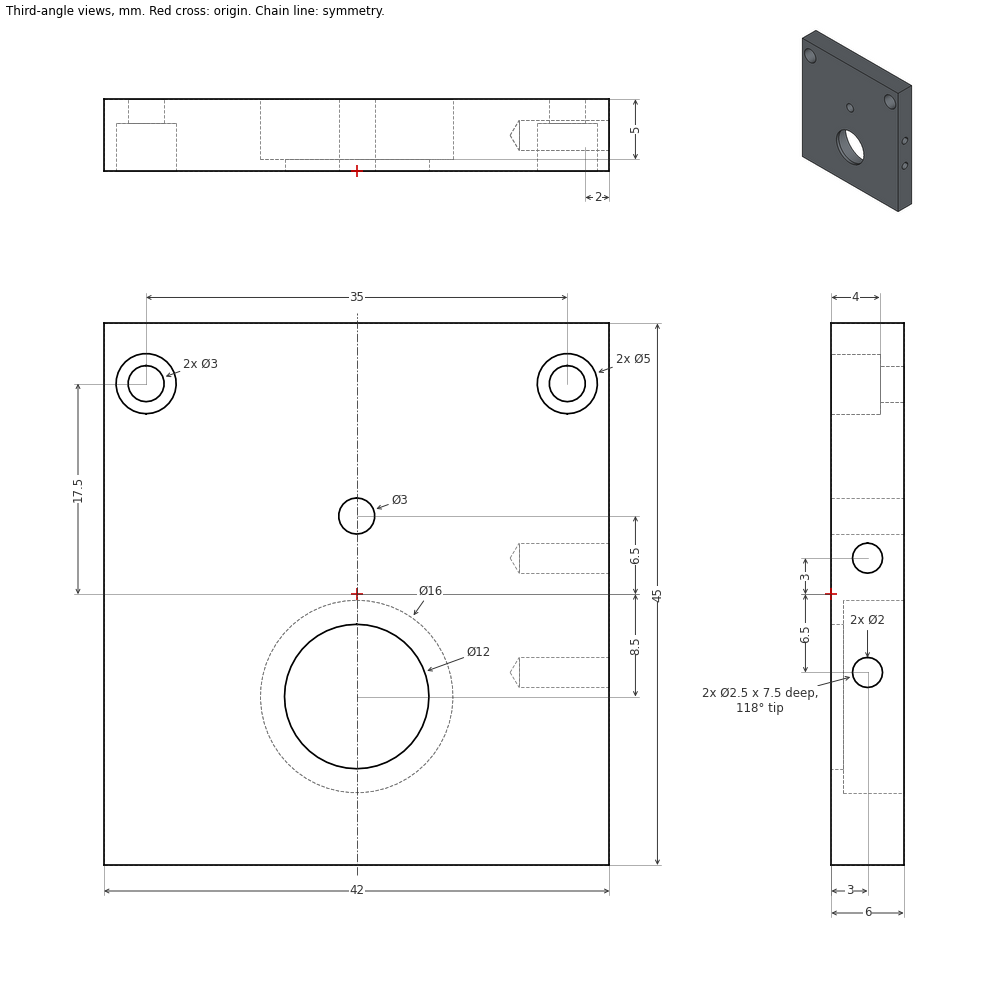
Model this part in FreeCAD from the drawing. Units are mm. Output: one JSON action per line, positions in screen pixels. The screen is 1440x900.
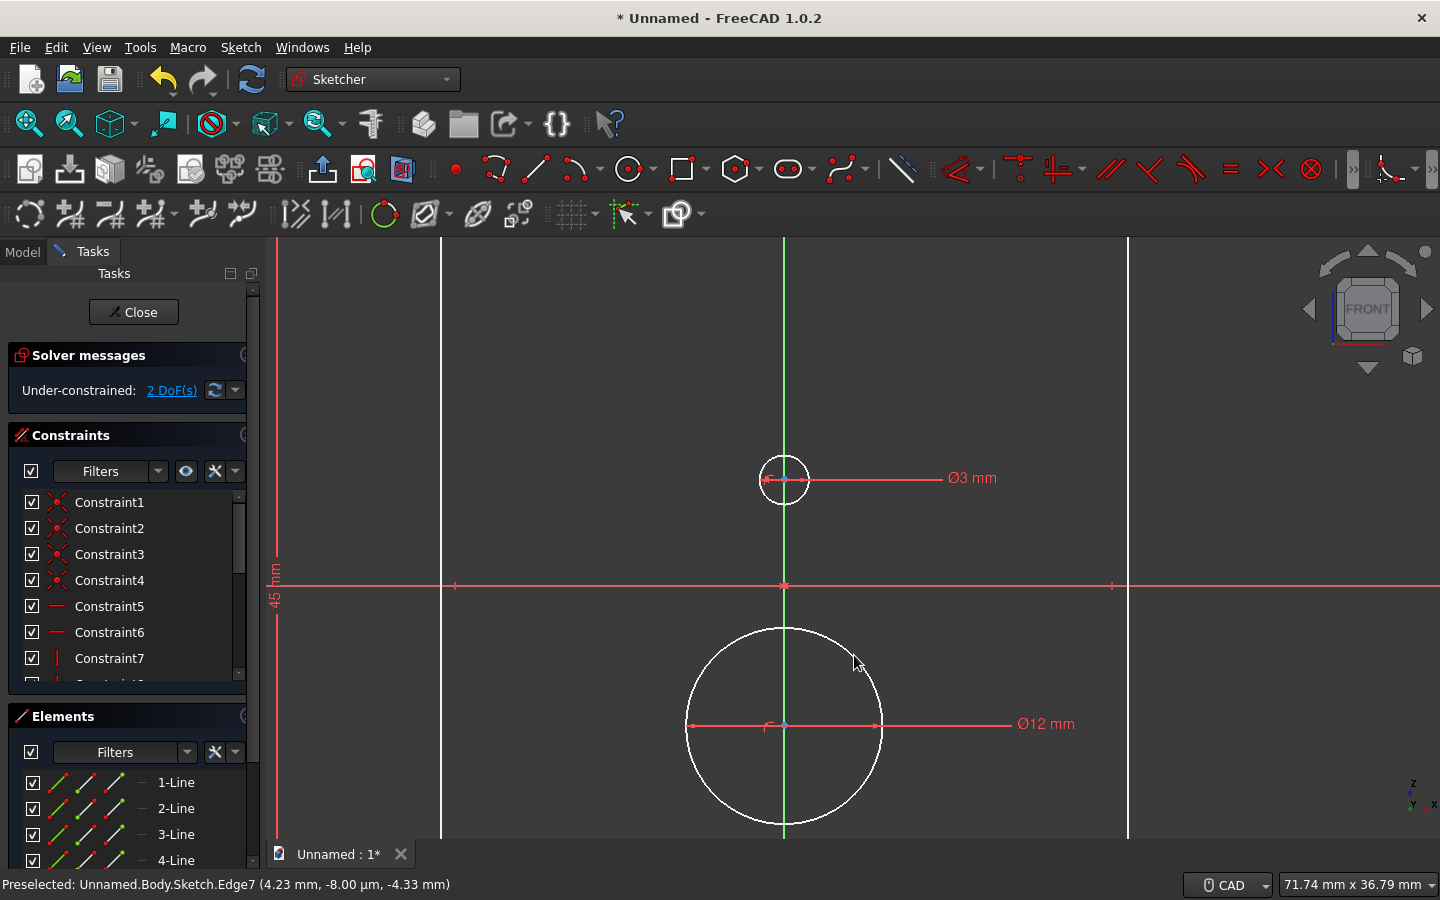
{"action": "key", "text": "d"}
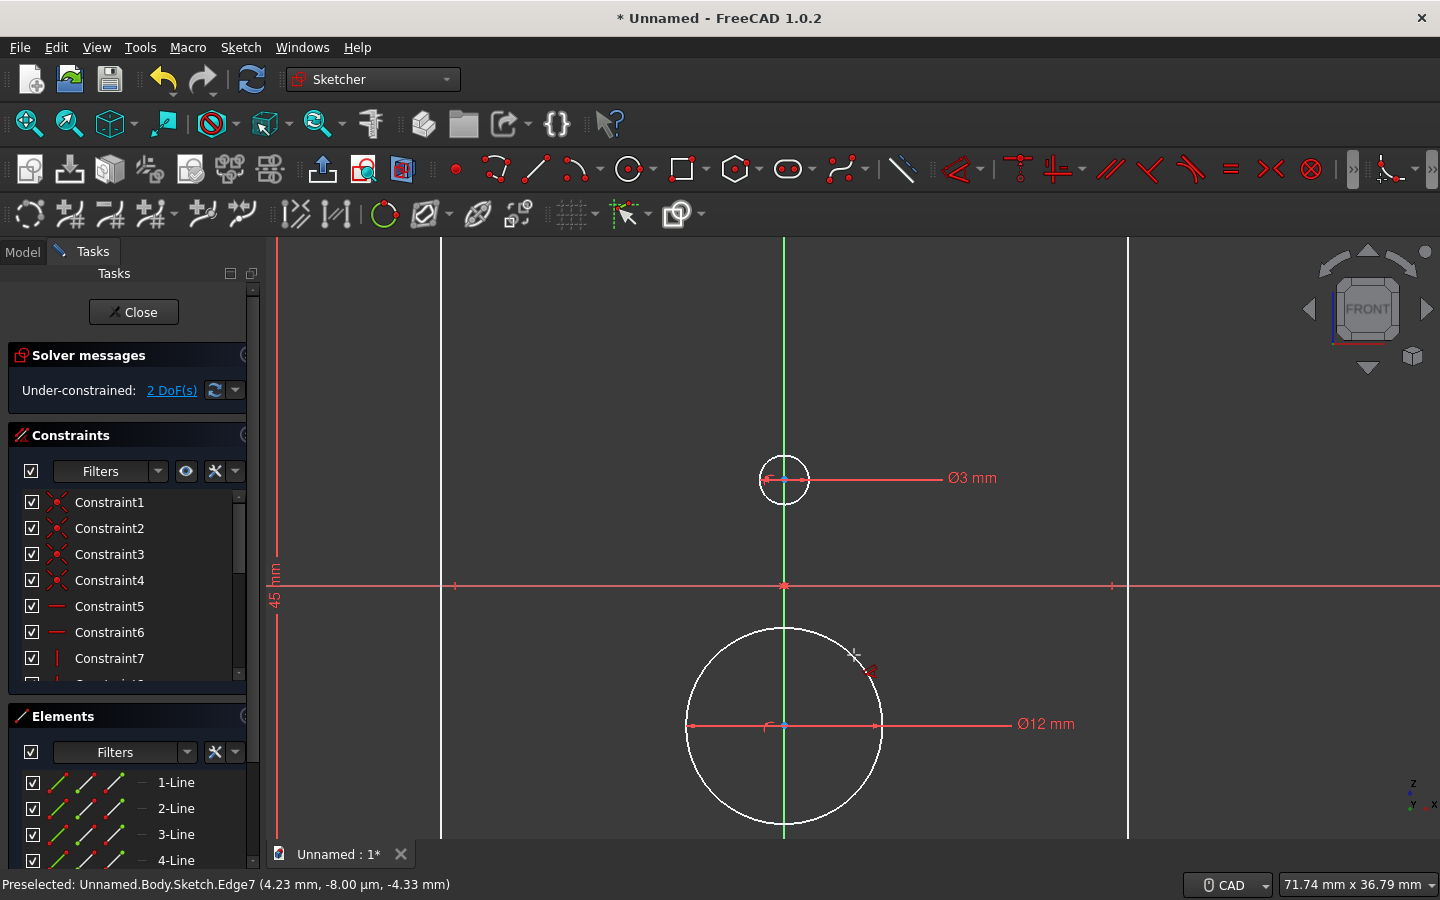
{"action": "left_click", "coordinate": [784, 480]}
{"action": "left_click", "coordinate": [818, 533]}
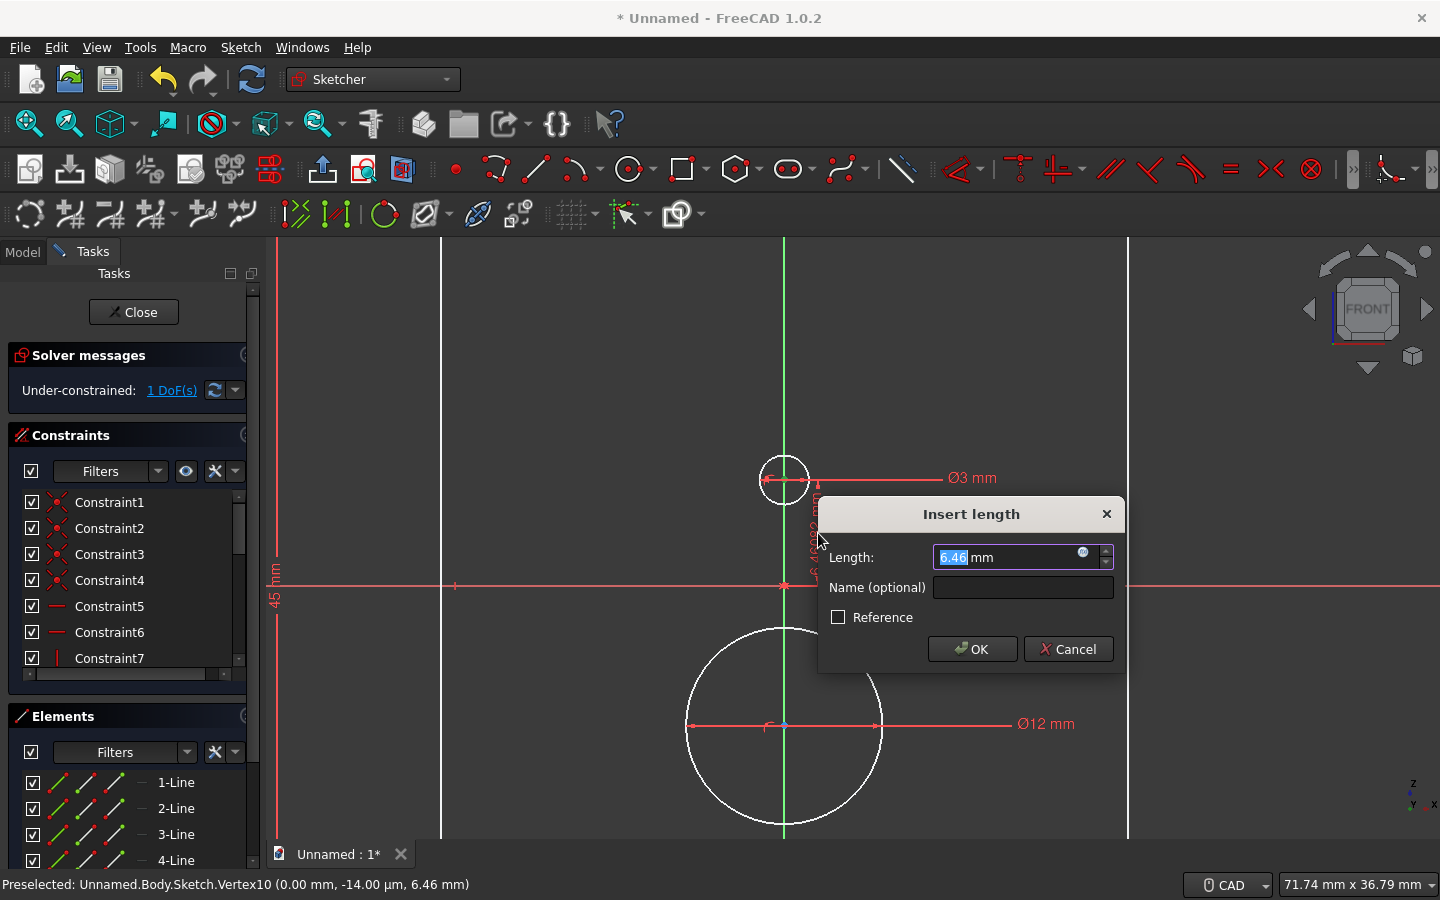
{"action": "type", "text": "6.5"}
{"action": "key", "text": "Return"}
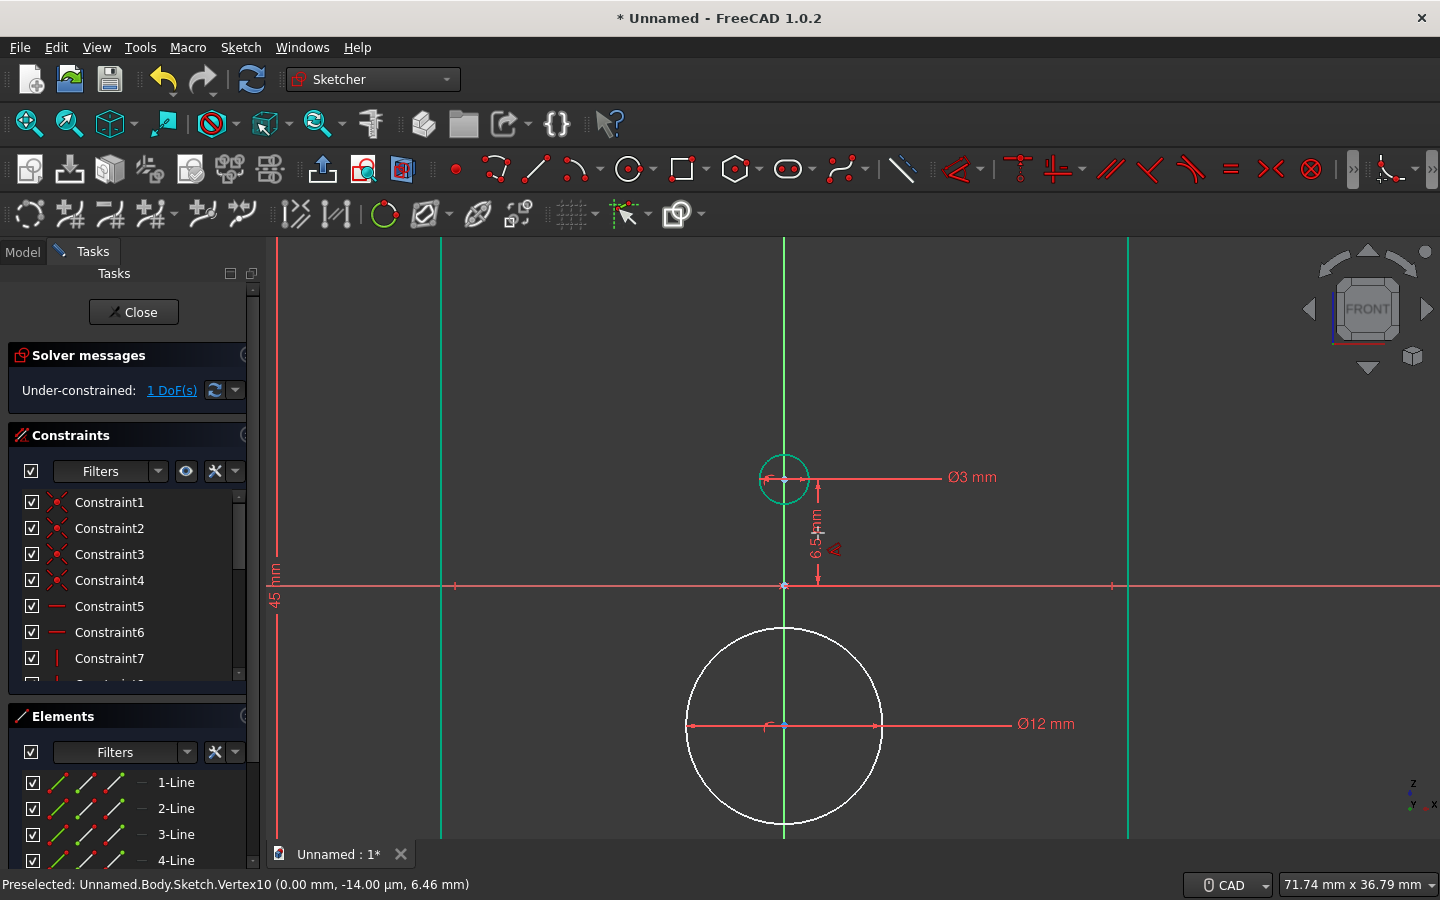
{"action": "left_click", "coordinate": [784, 726]}
{"action": "left_click", "coordinate": [818, 656]}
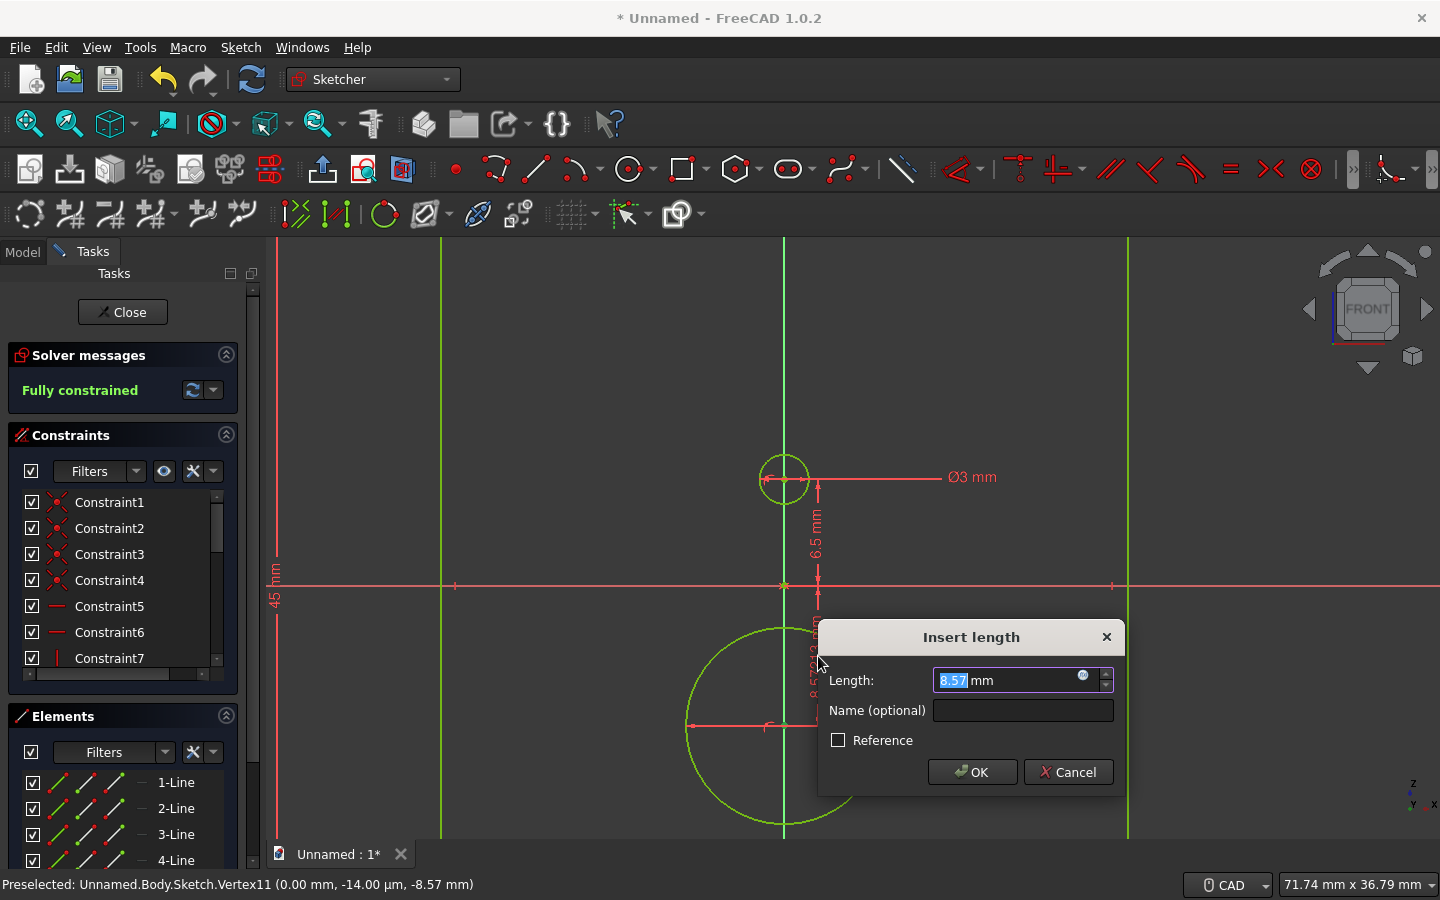
{"action": "type", "text": "8.5"}
{"action": "key", "text": "Return"}
{"action": "key", "text": "Escape"}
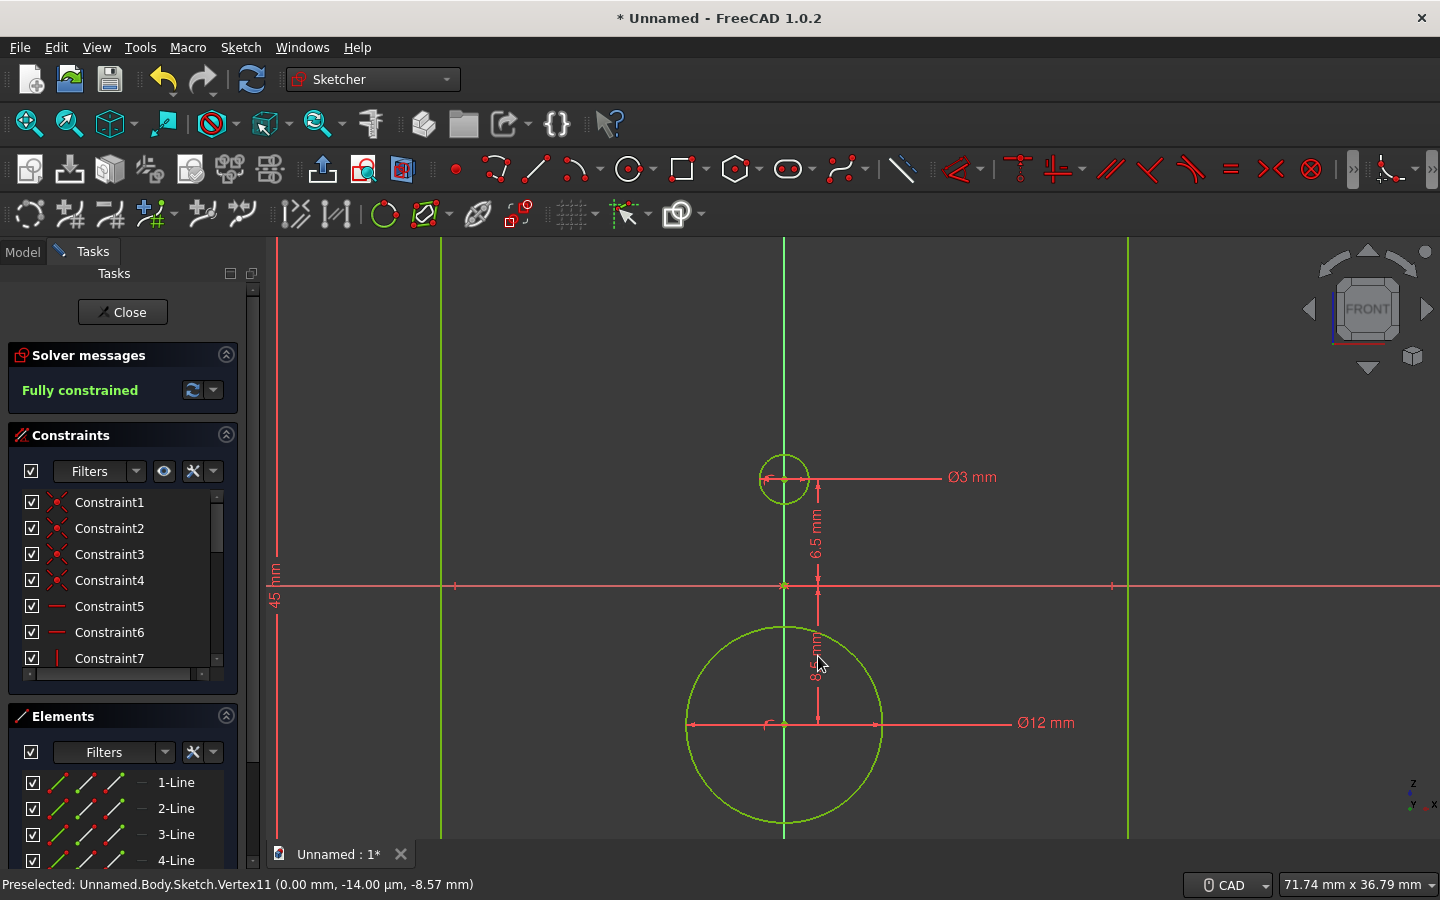
{"action": "left_click", "coordinate": [123, 312]}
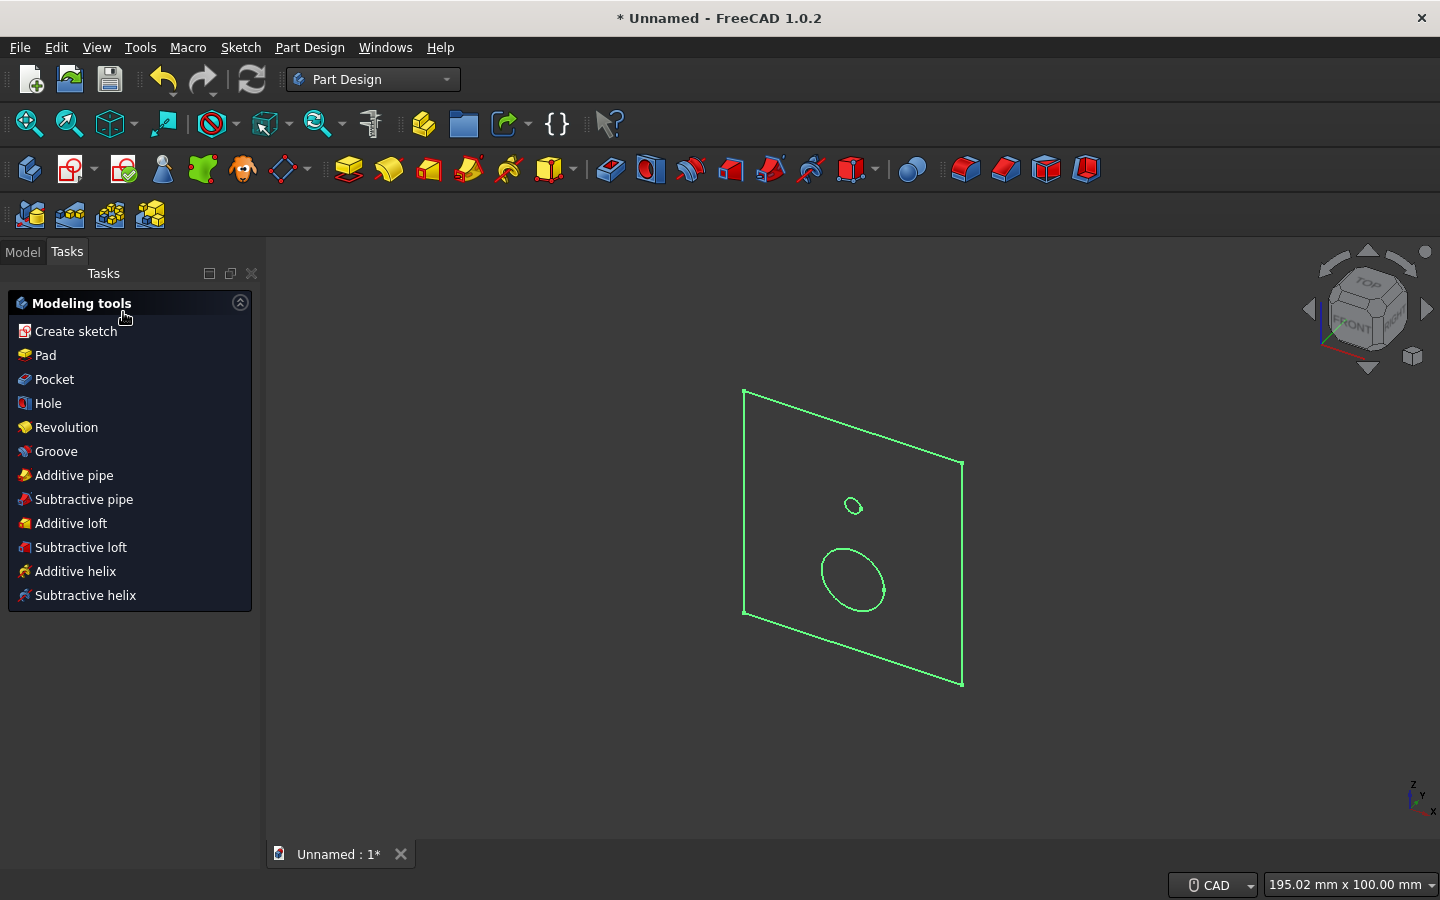
{"action": "left_click", "coordinate": [350, 170]}